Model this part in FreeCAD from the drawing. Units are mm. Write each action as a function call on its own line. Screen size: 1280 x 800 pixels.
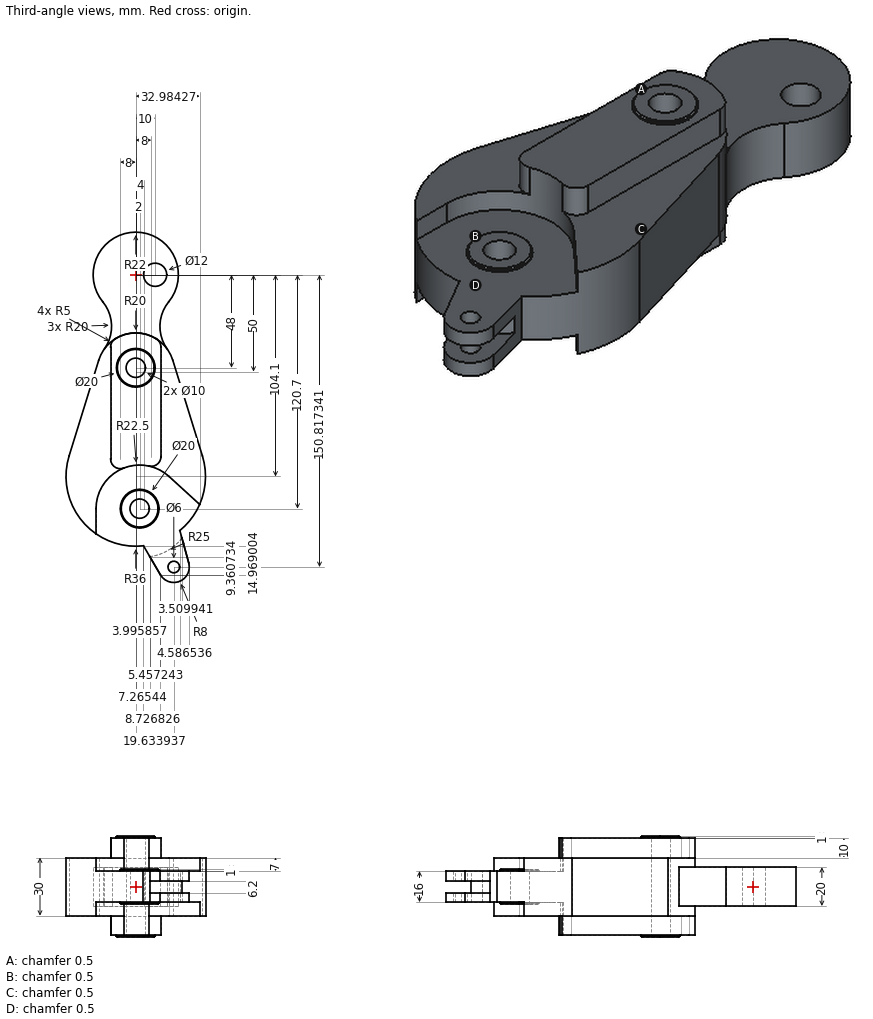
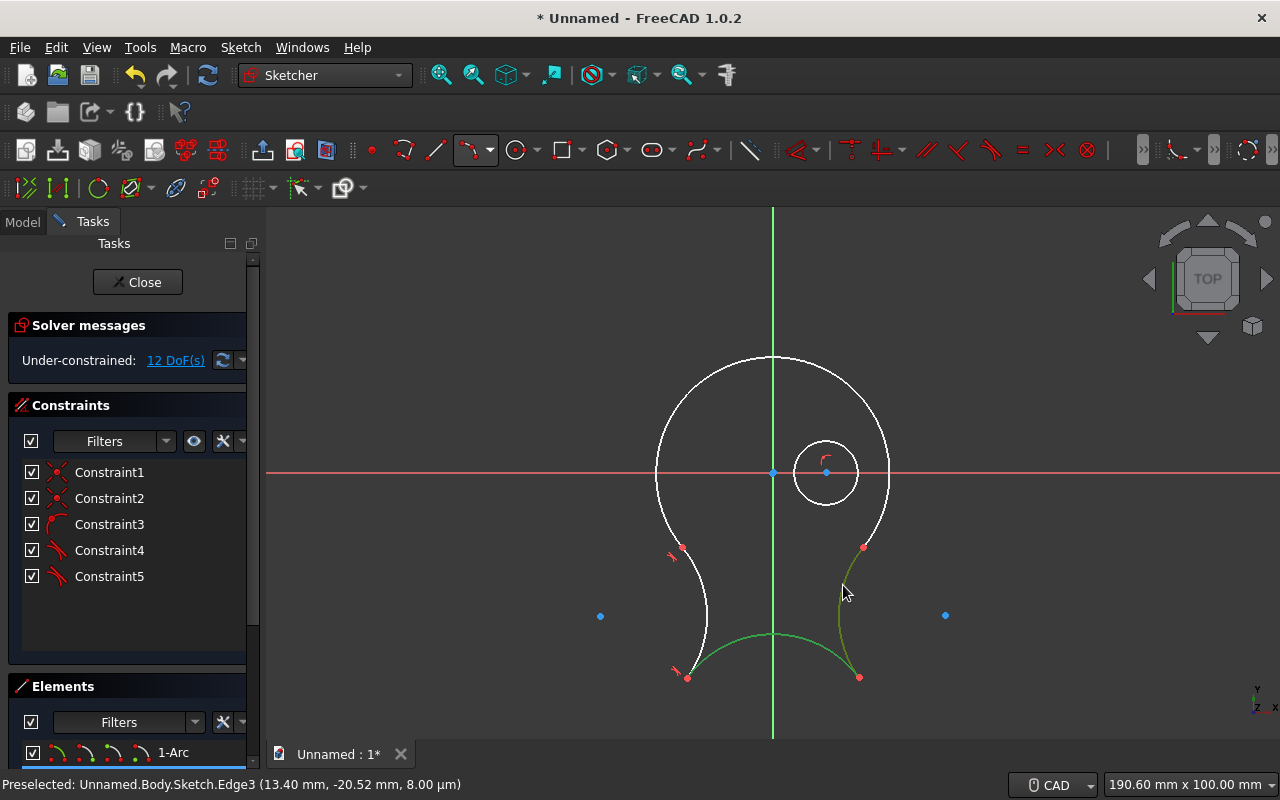
click(992, 150)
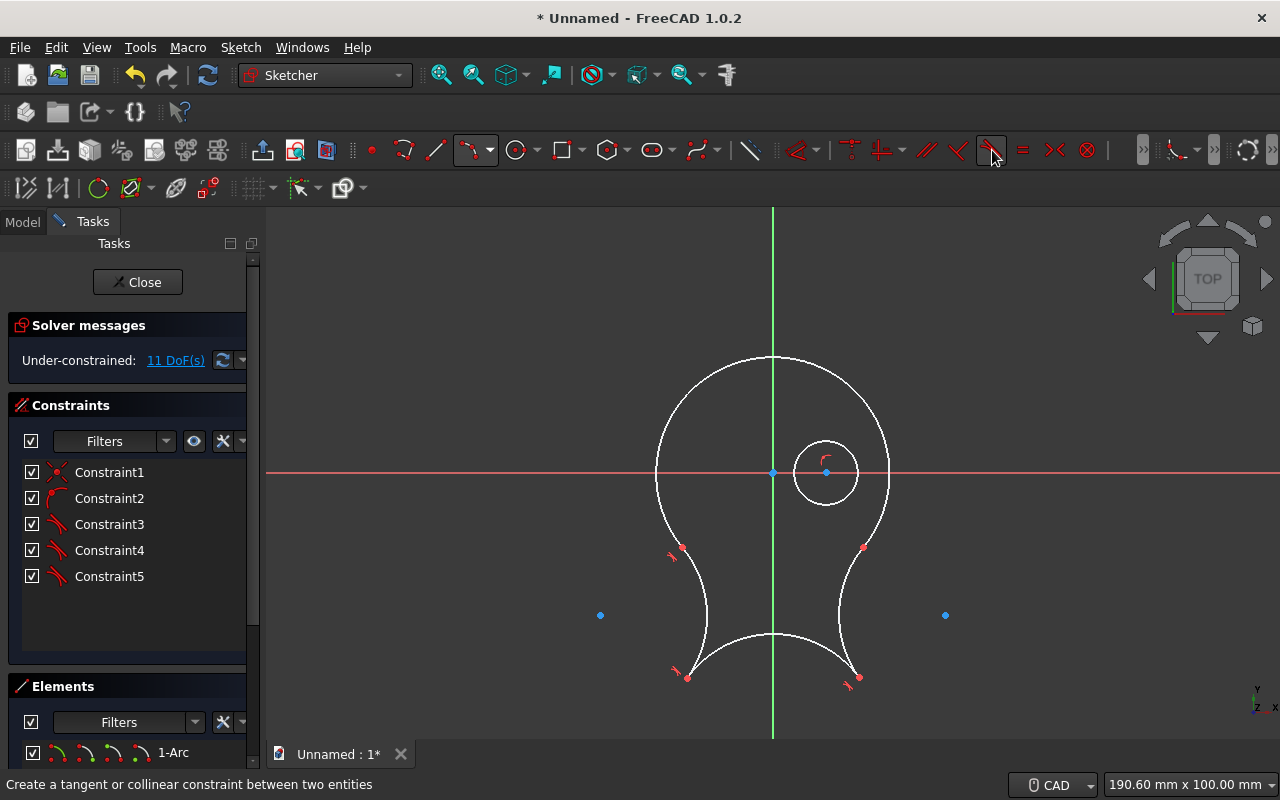
click(844, 585)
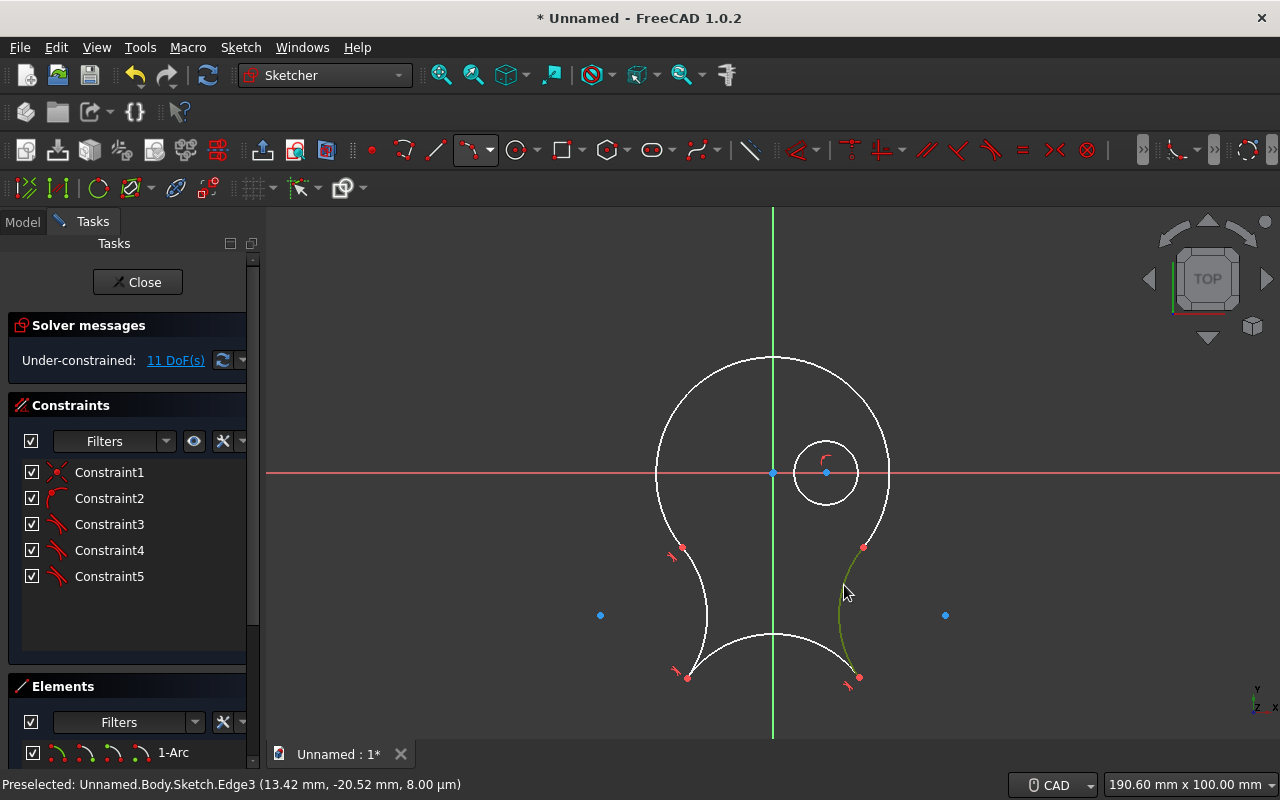
click(865, 402)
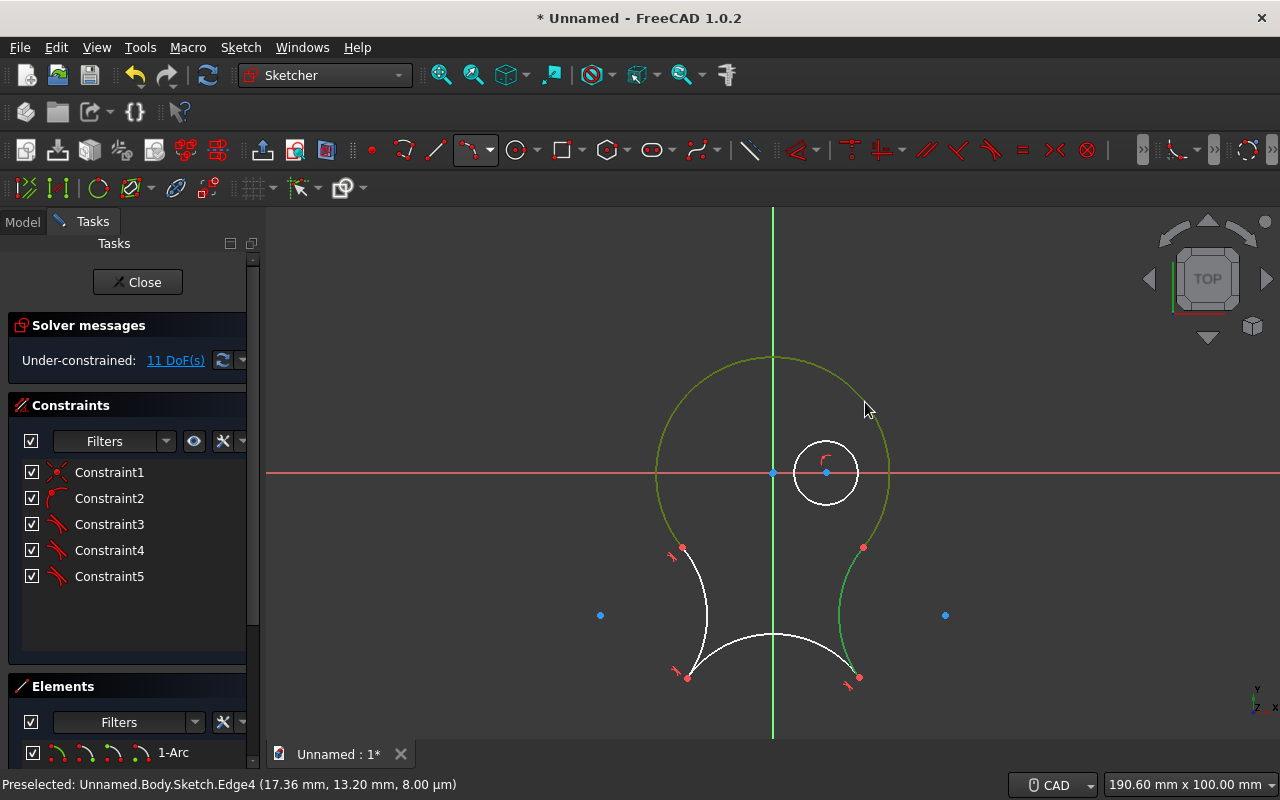
click(992, 150)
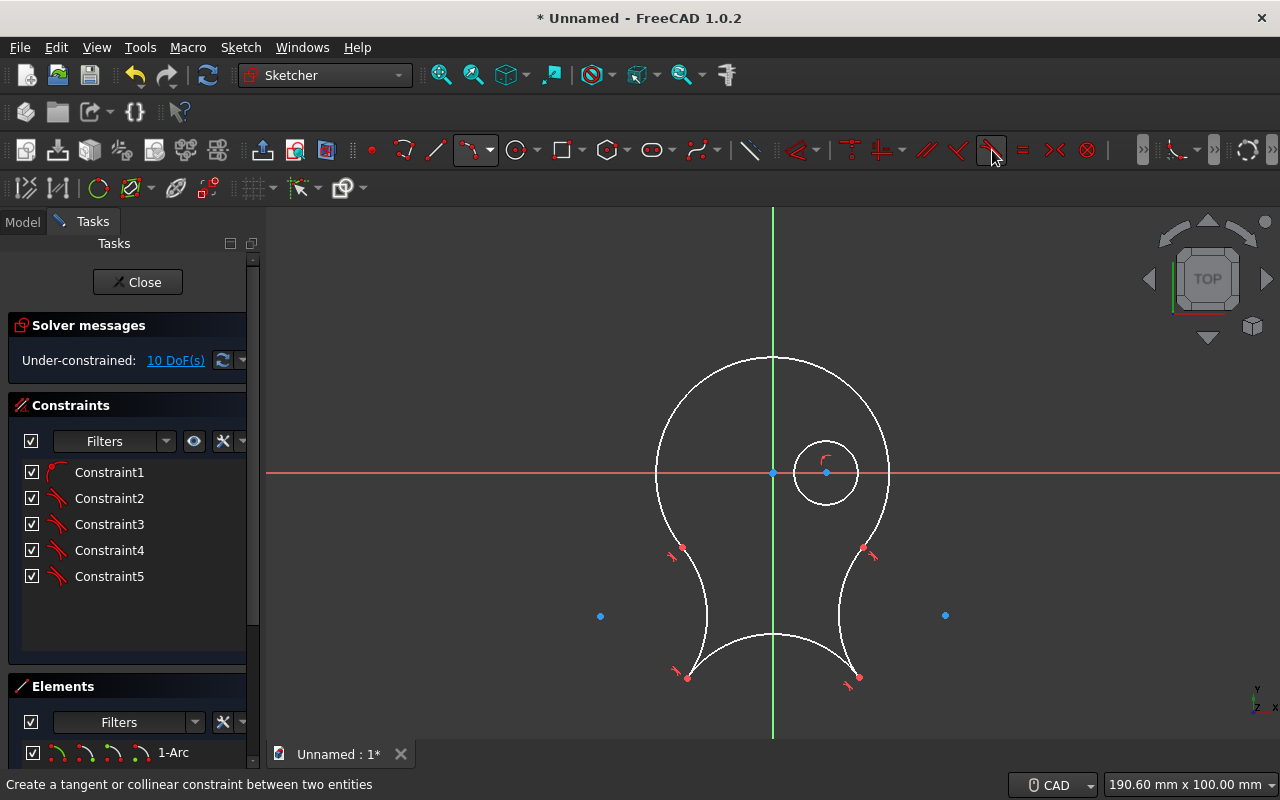
scroll(773, 473, up, 2)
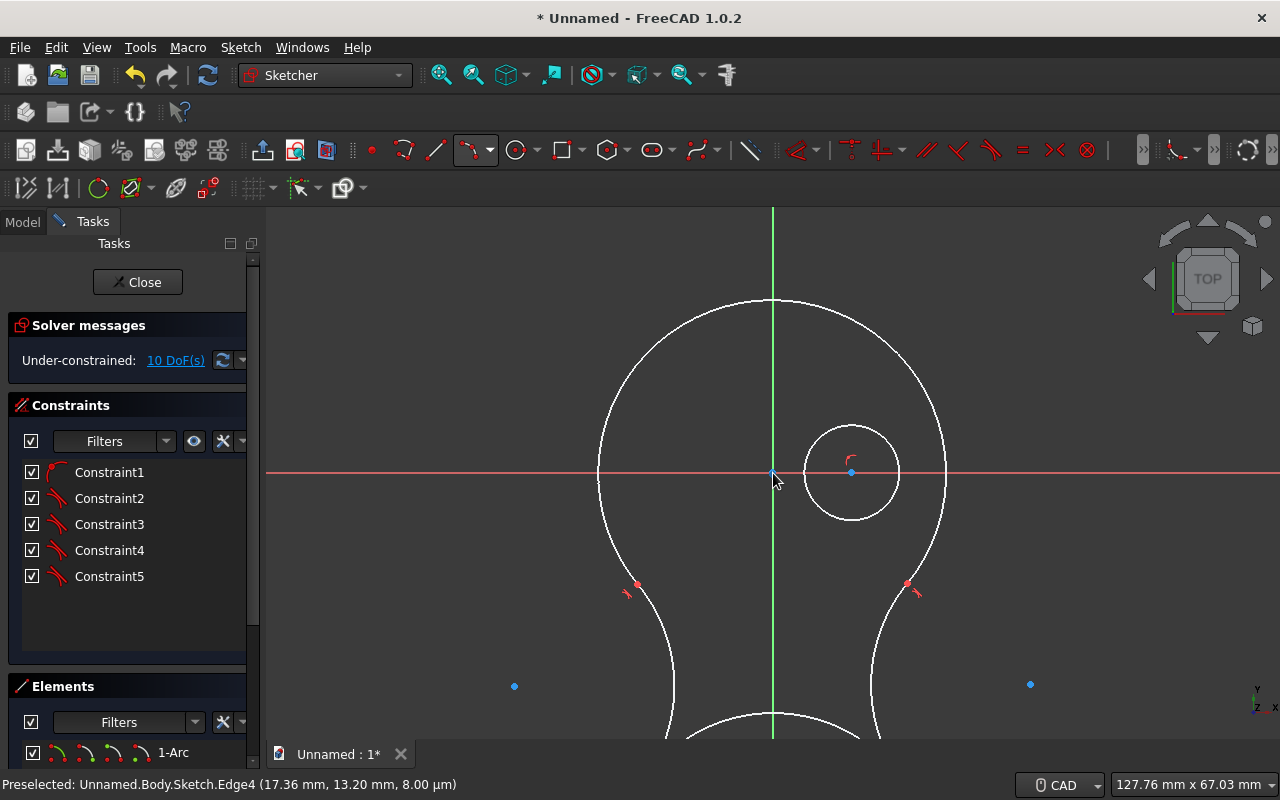
drag(762, 463, 783, 484)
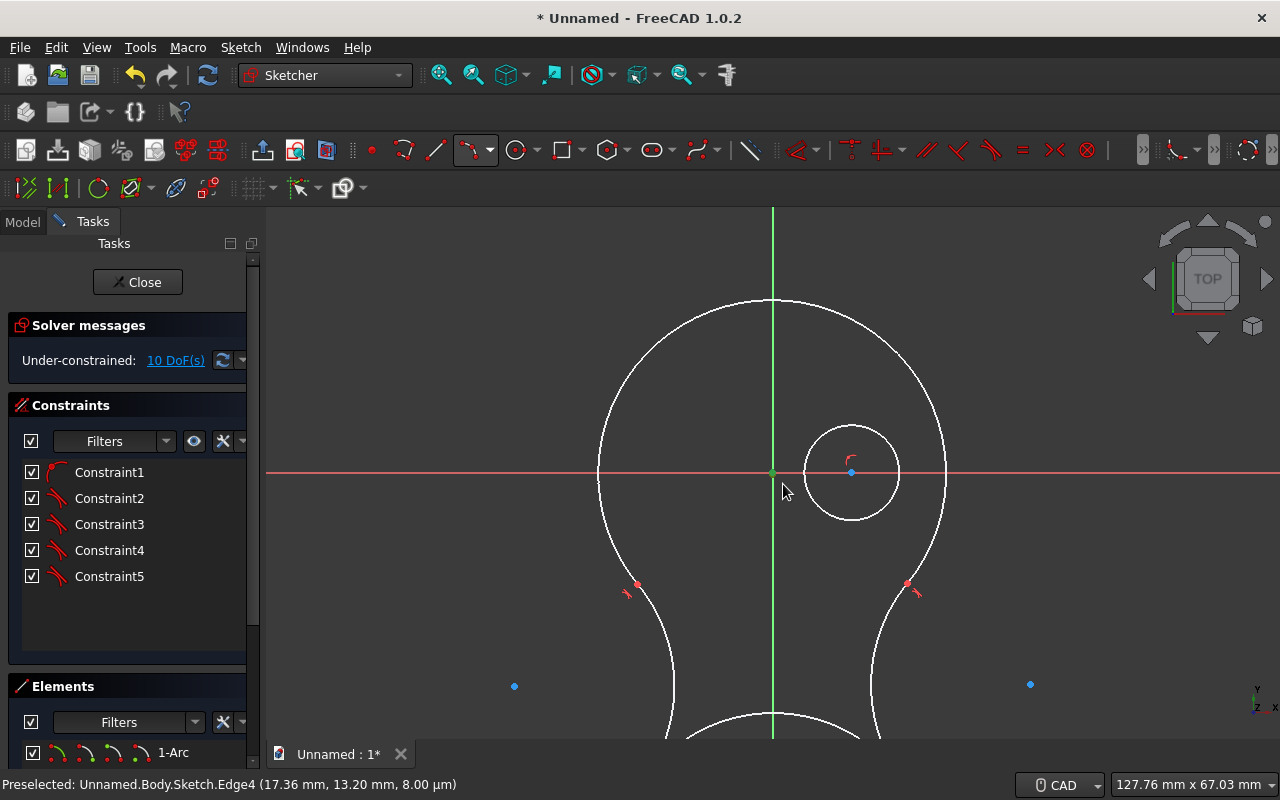
click(850, 150)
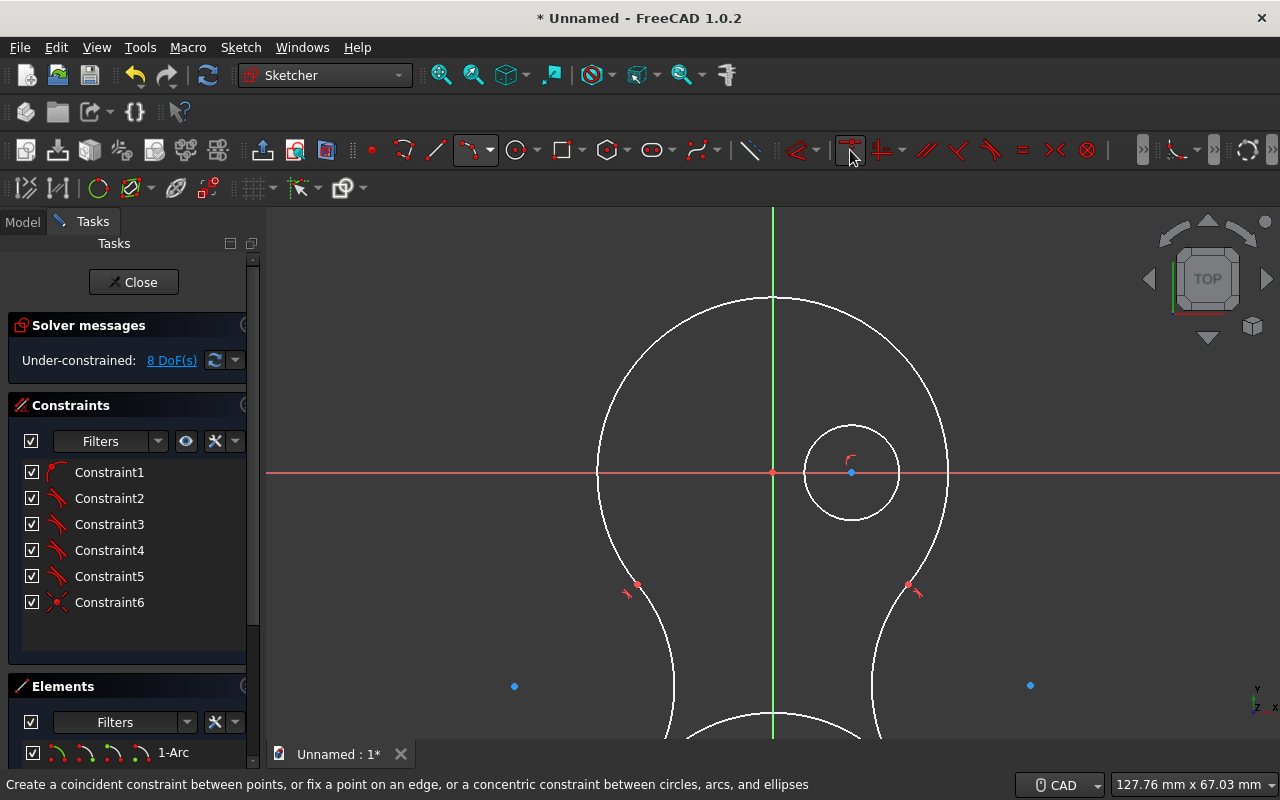
click(667, 640)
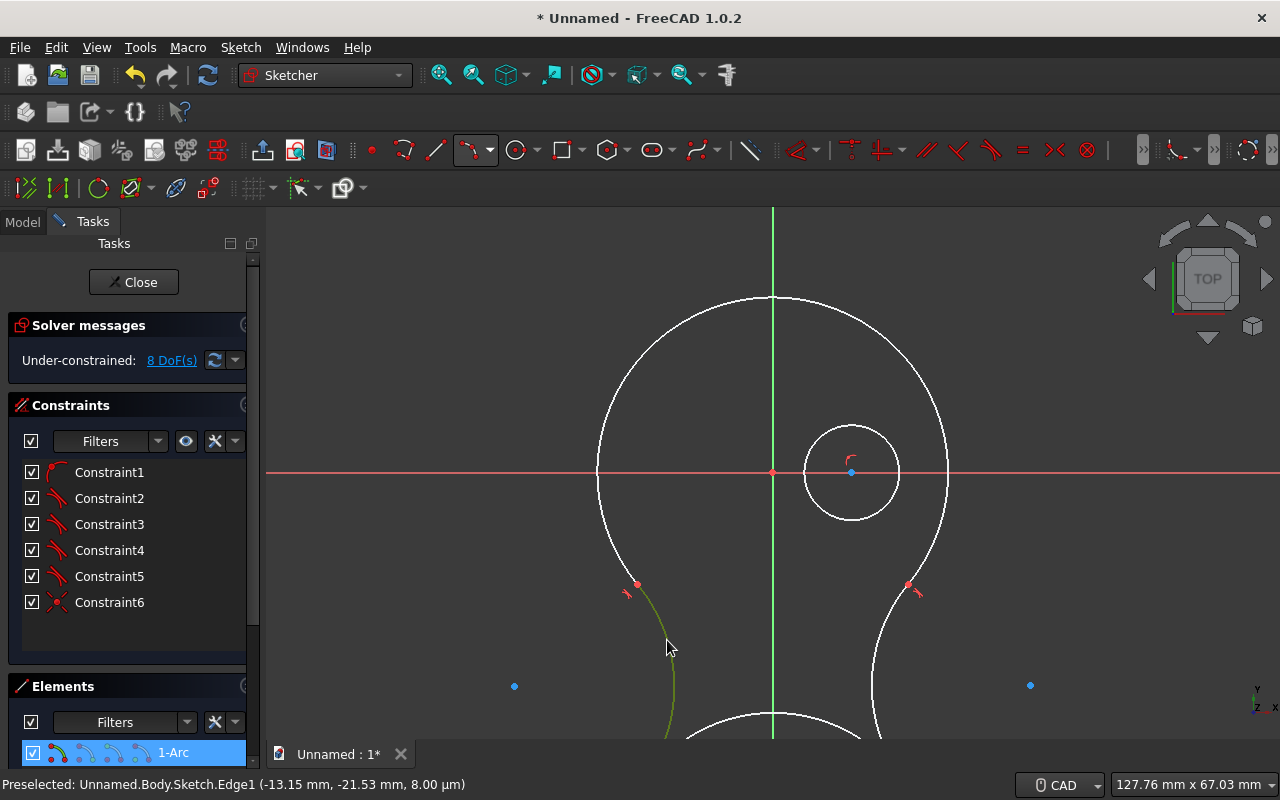
scroll(566, 342, down, 2)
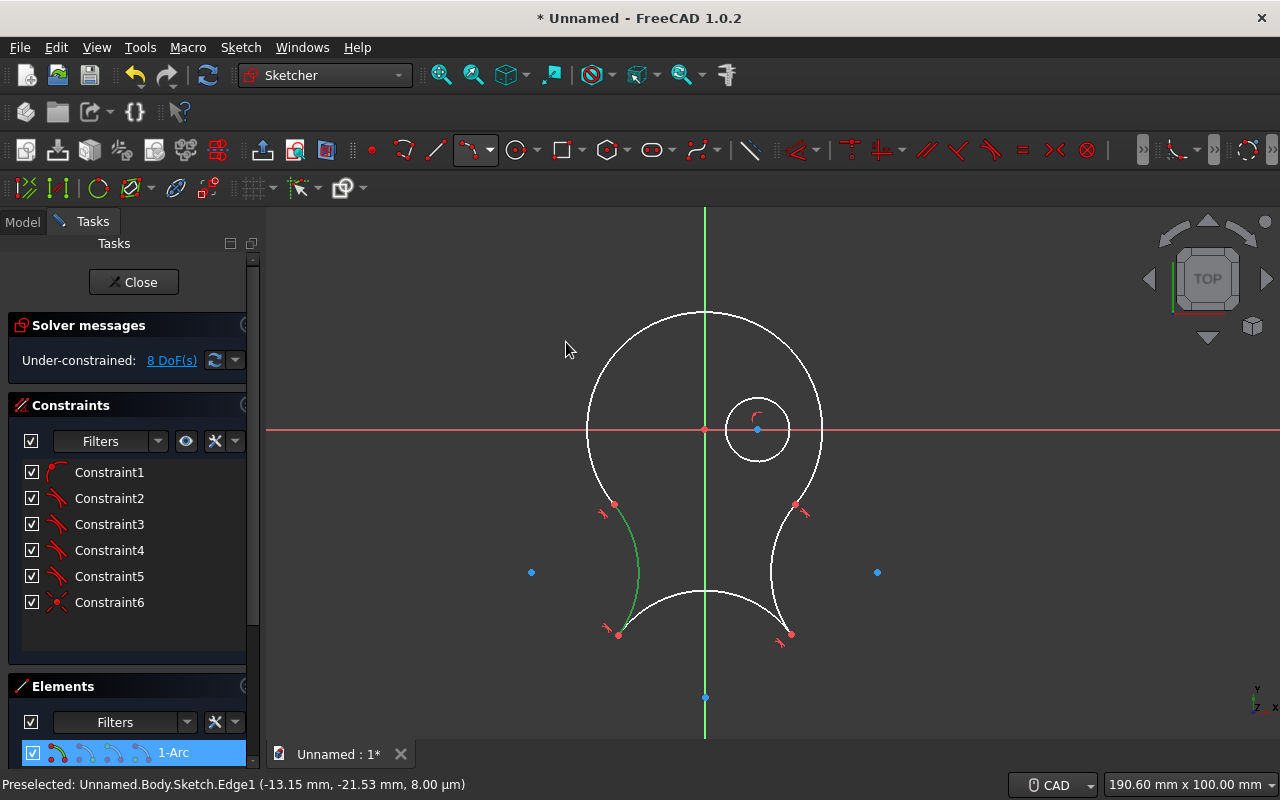
click(744, 598)